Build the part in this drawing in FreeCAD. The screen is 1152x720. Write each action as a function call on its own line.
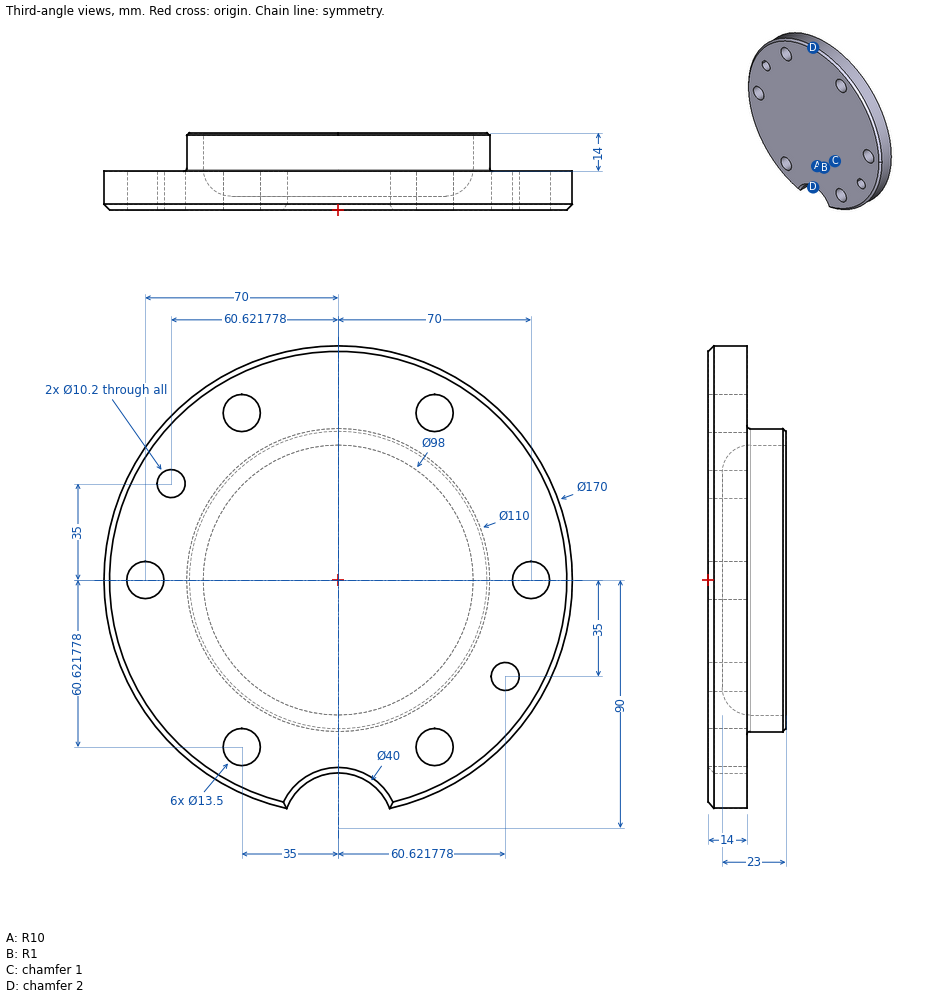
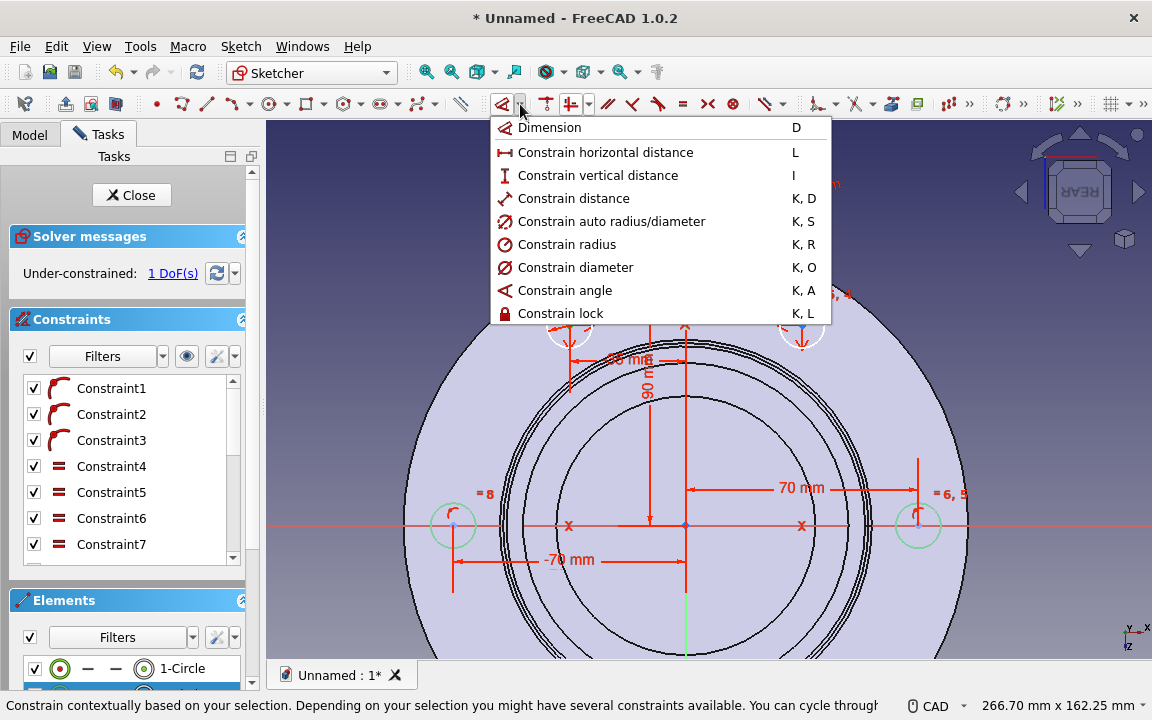
click(661, 176)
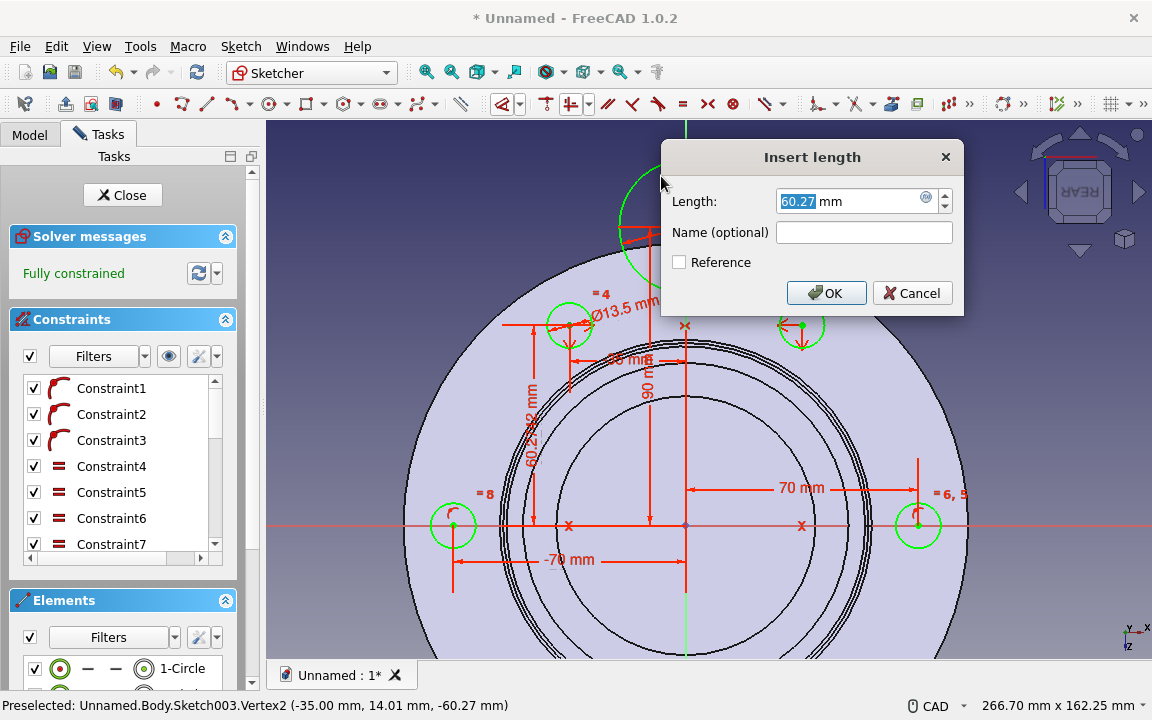
text(60.621778)
key(Return)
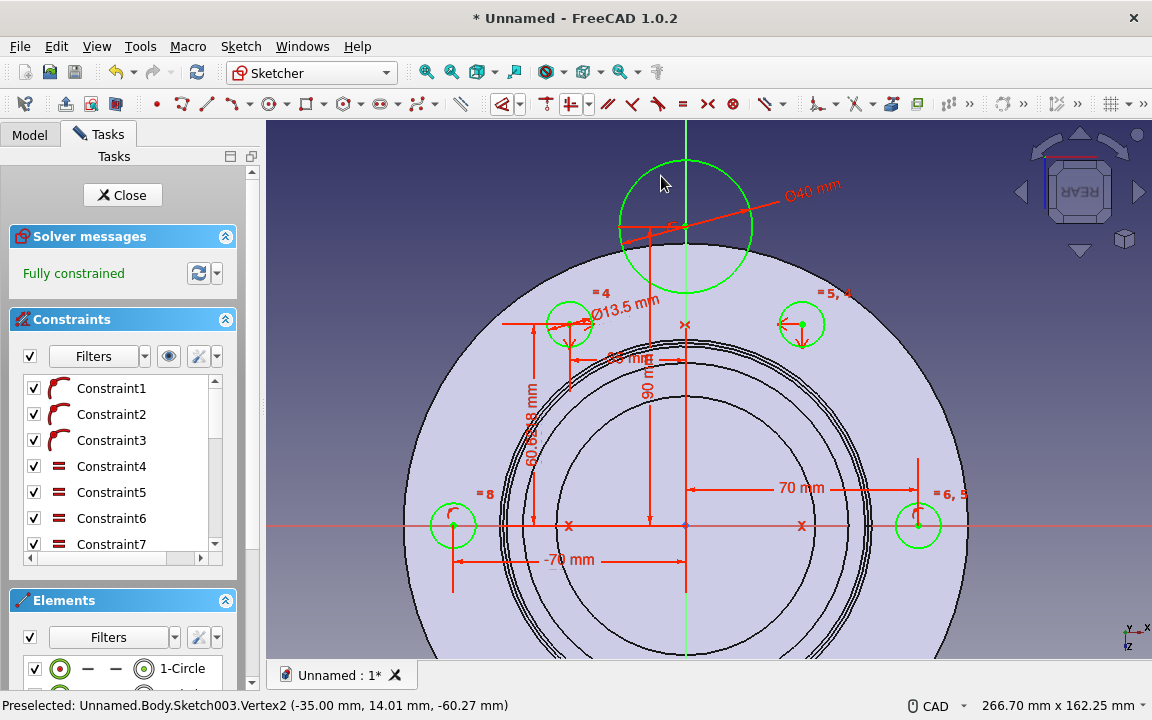
click(123, 195)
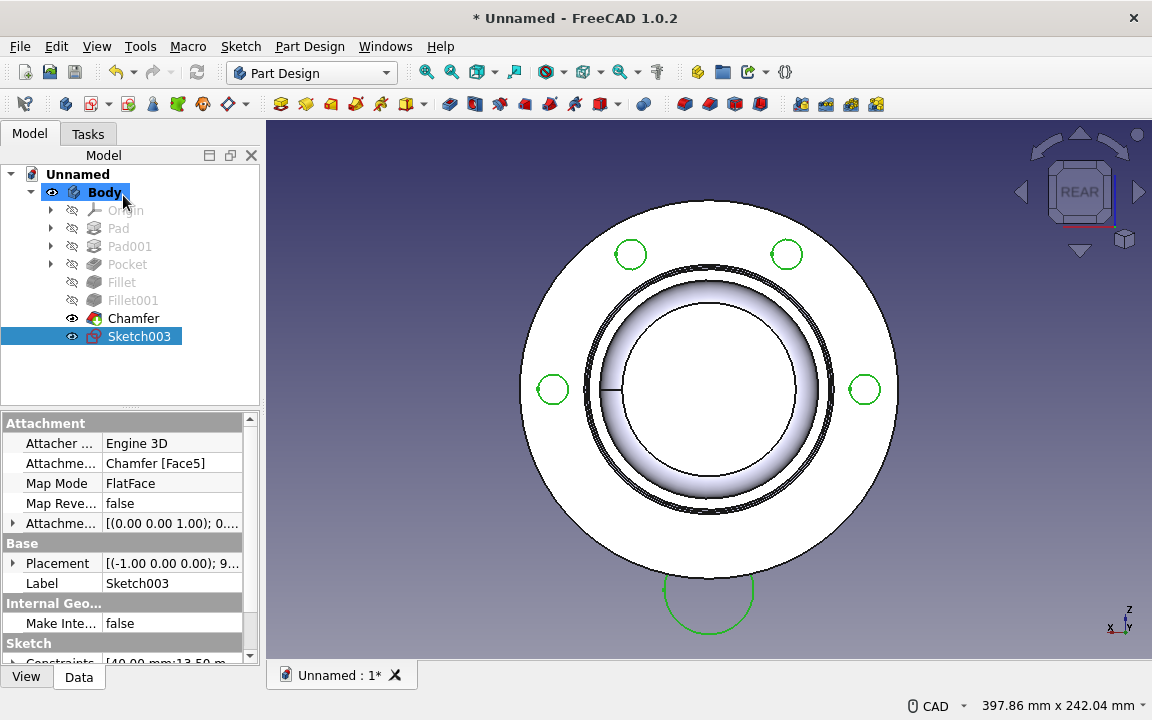
click(450, 104)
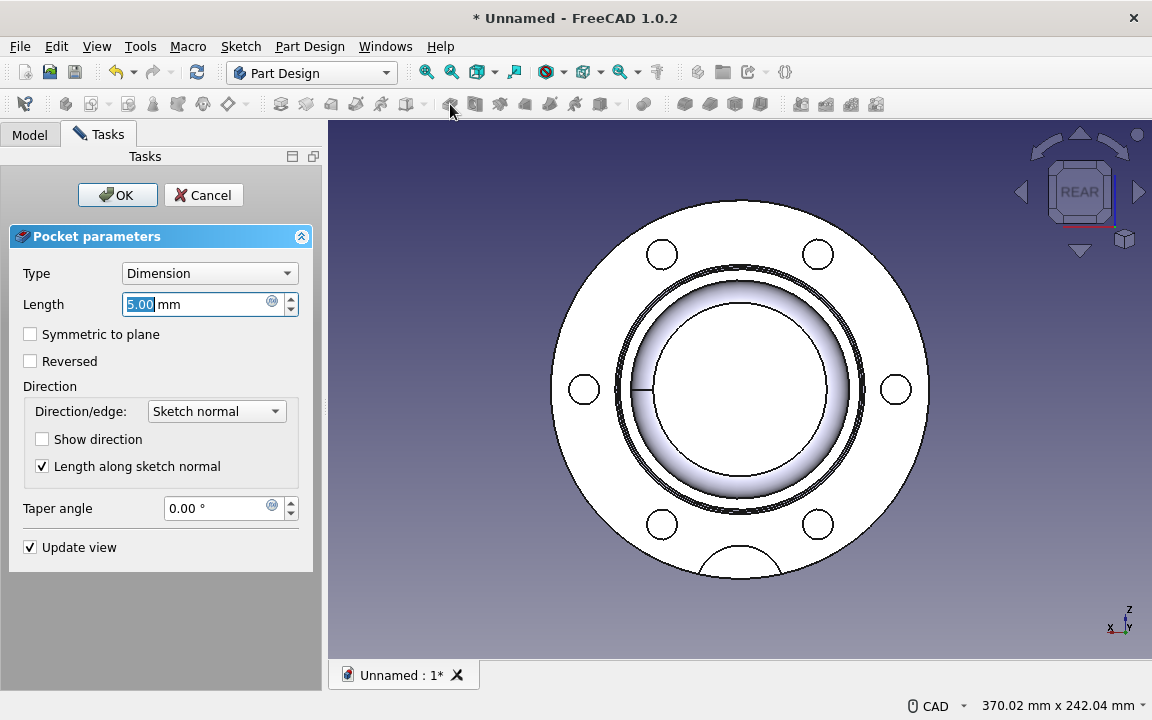
click(210, 274)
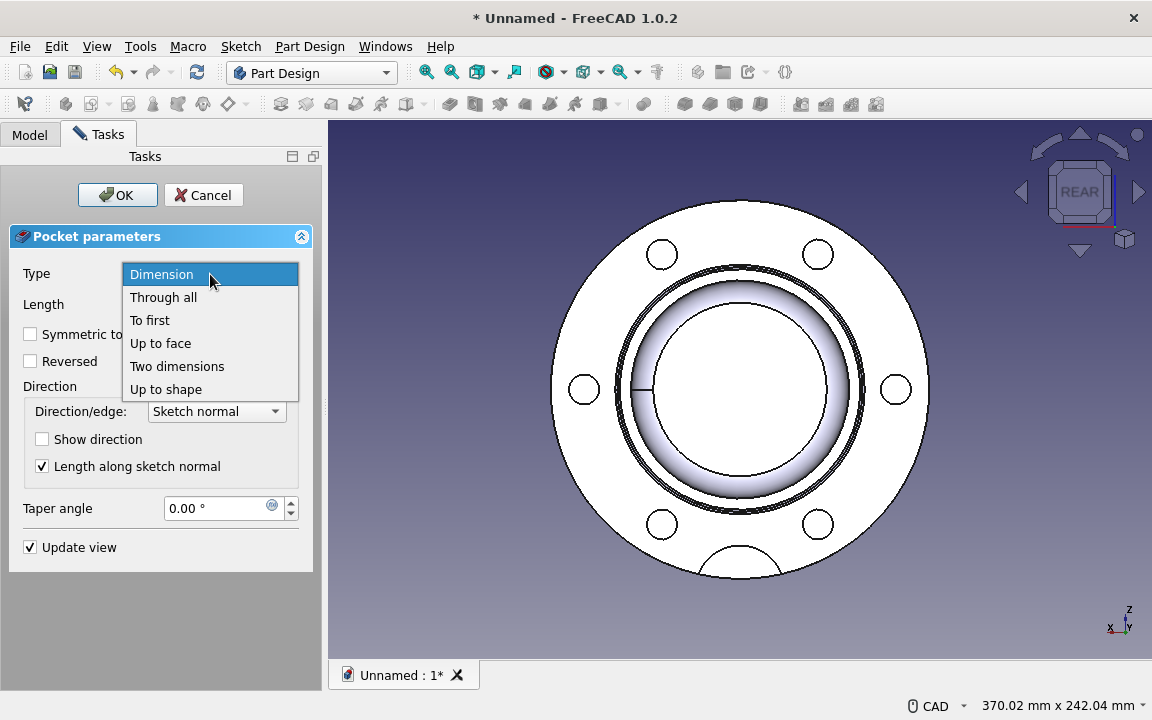
click(208, 298)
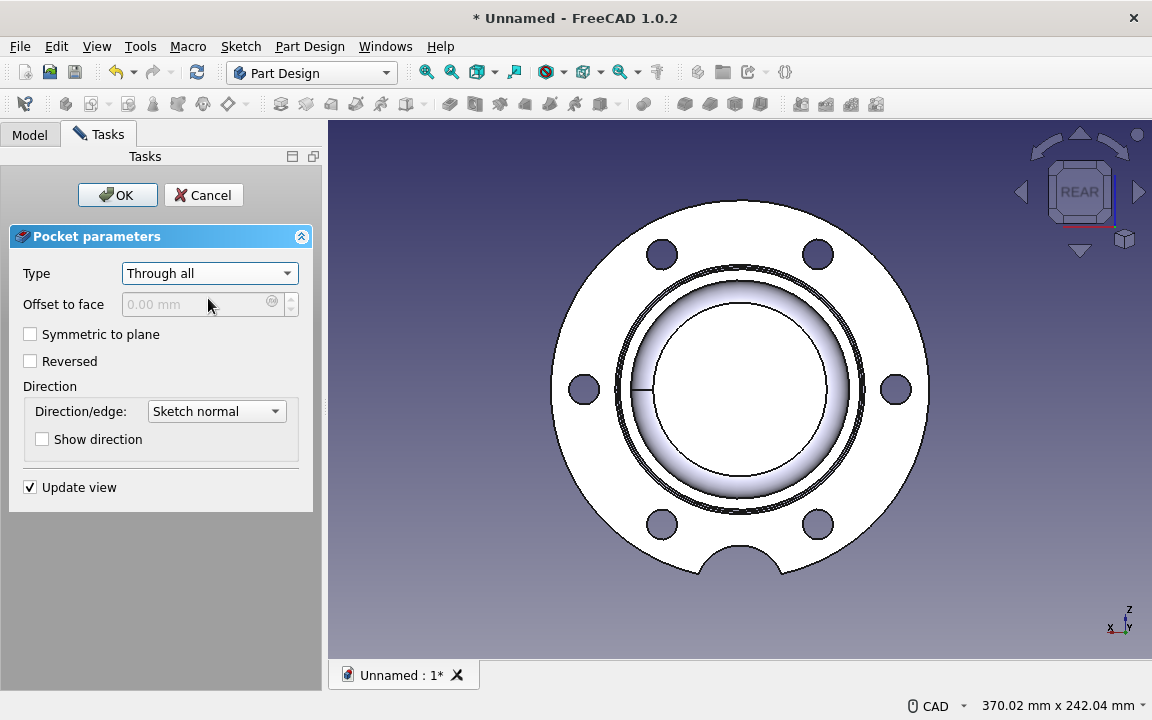
click(118, 195)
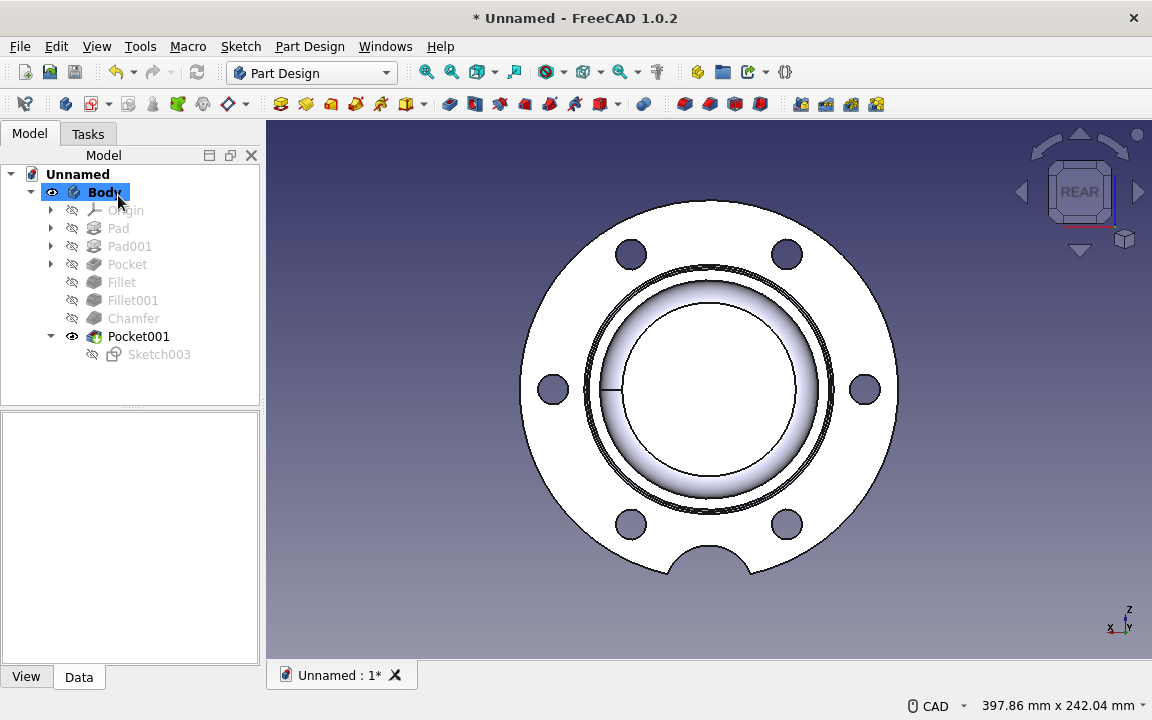
click(709, 226)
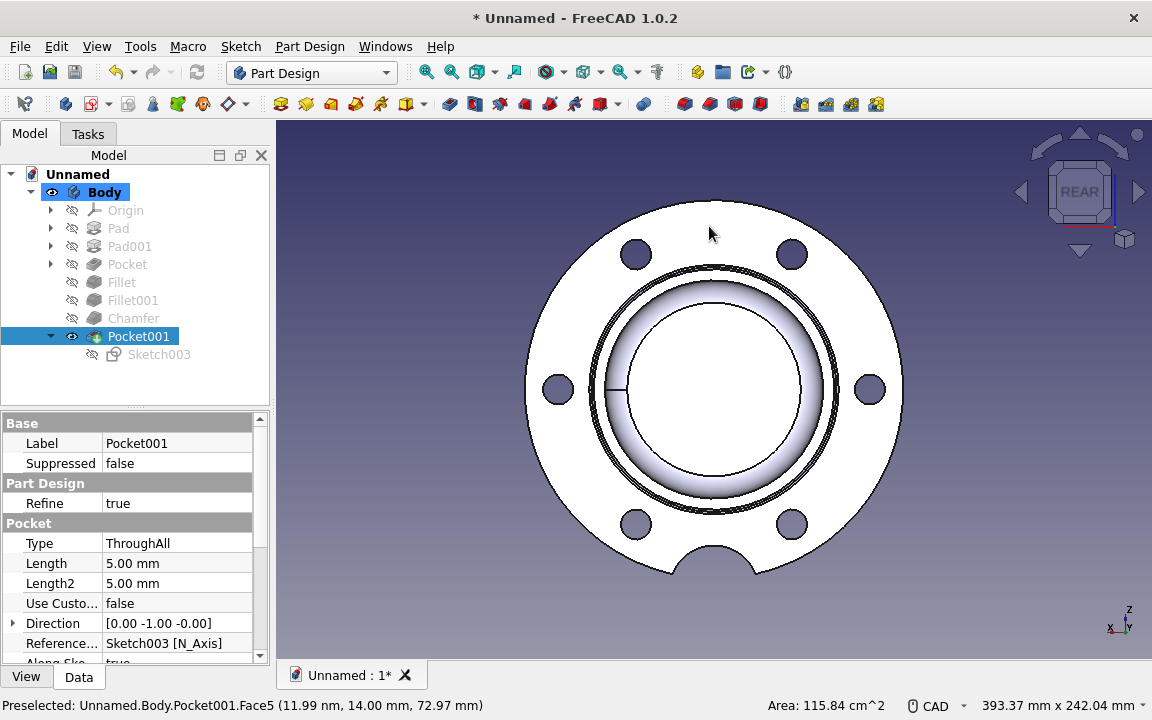
click(90, 104)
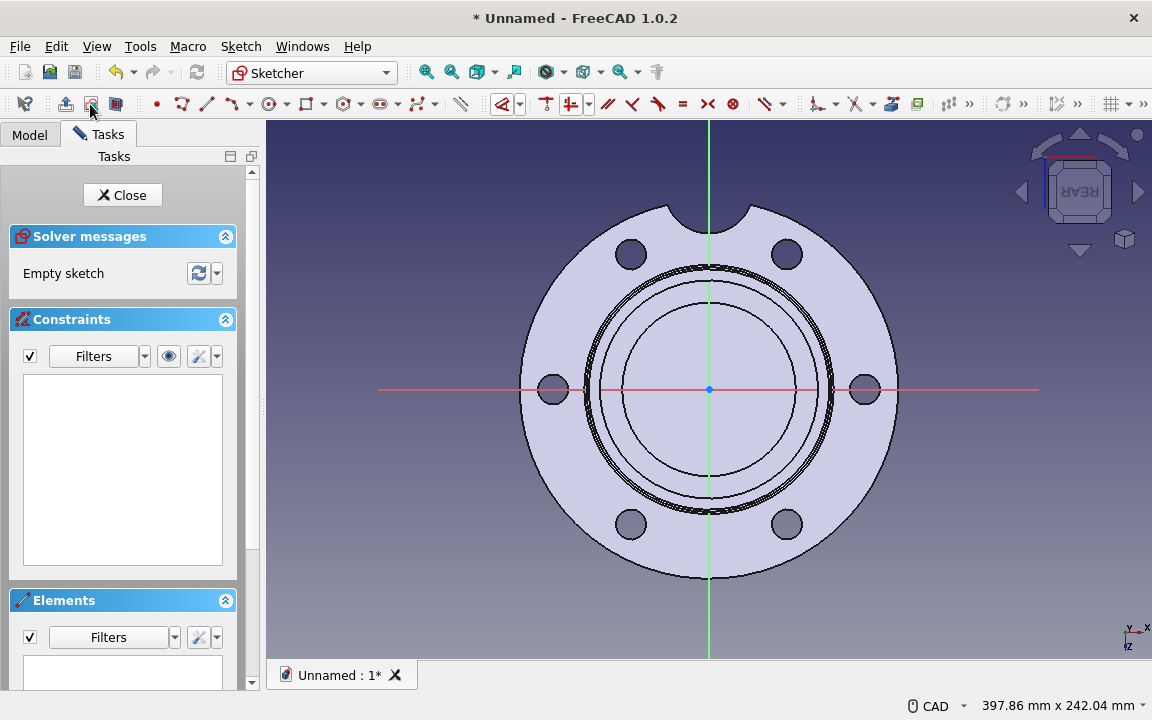
click(116, 104)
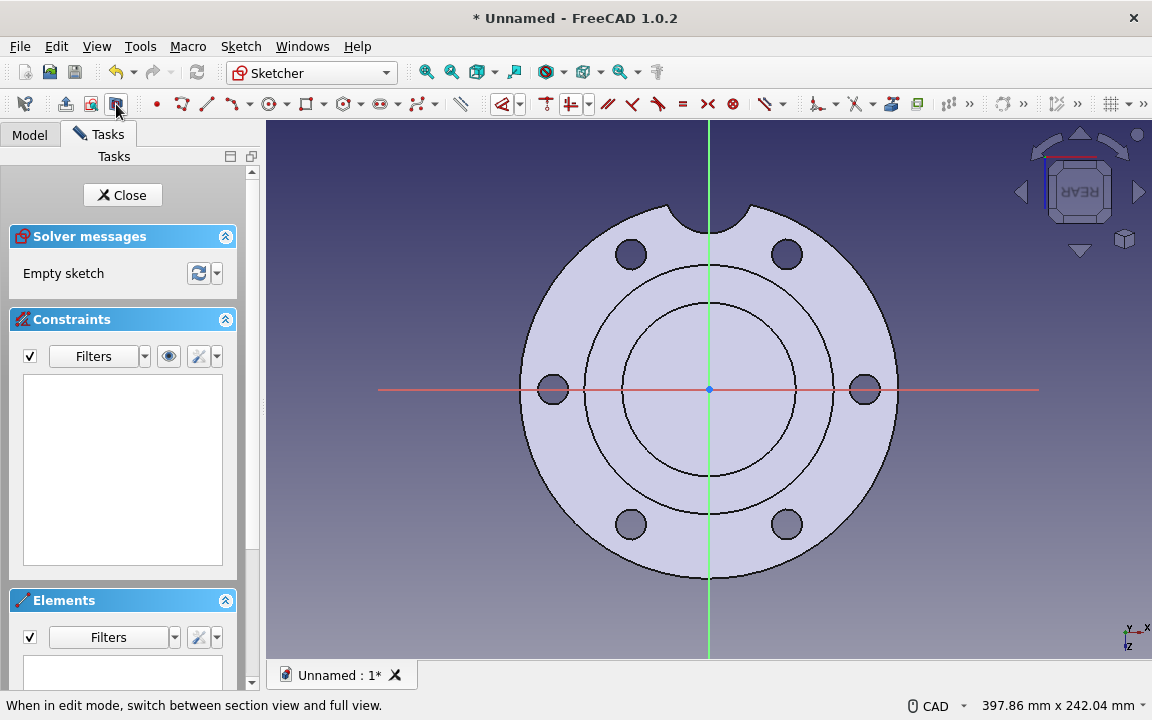
scroll(792, 389, up, 3)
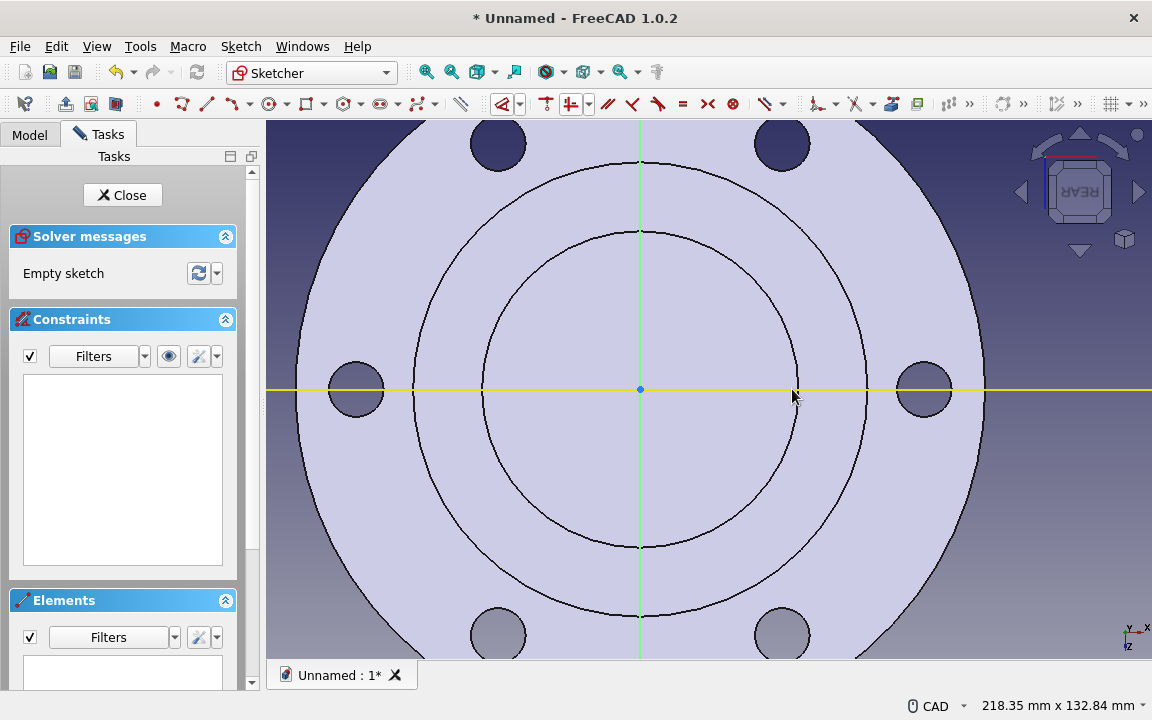
click(268, 104)